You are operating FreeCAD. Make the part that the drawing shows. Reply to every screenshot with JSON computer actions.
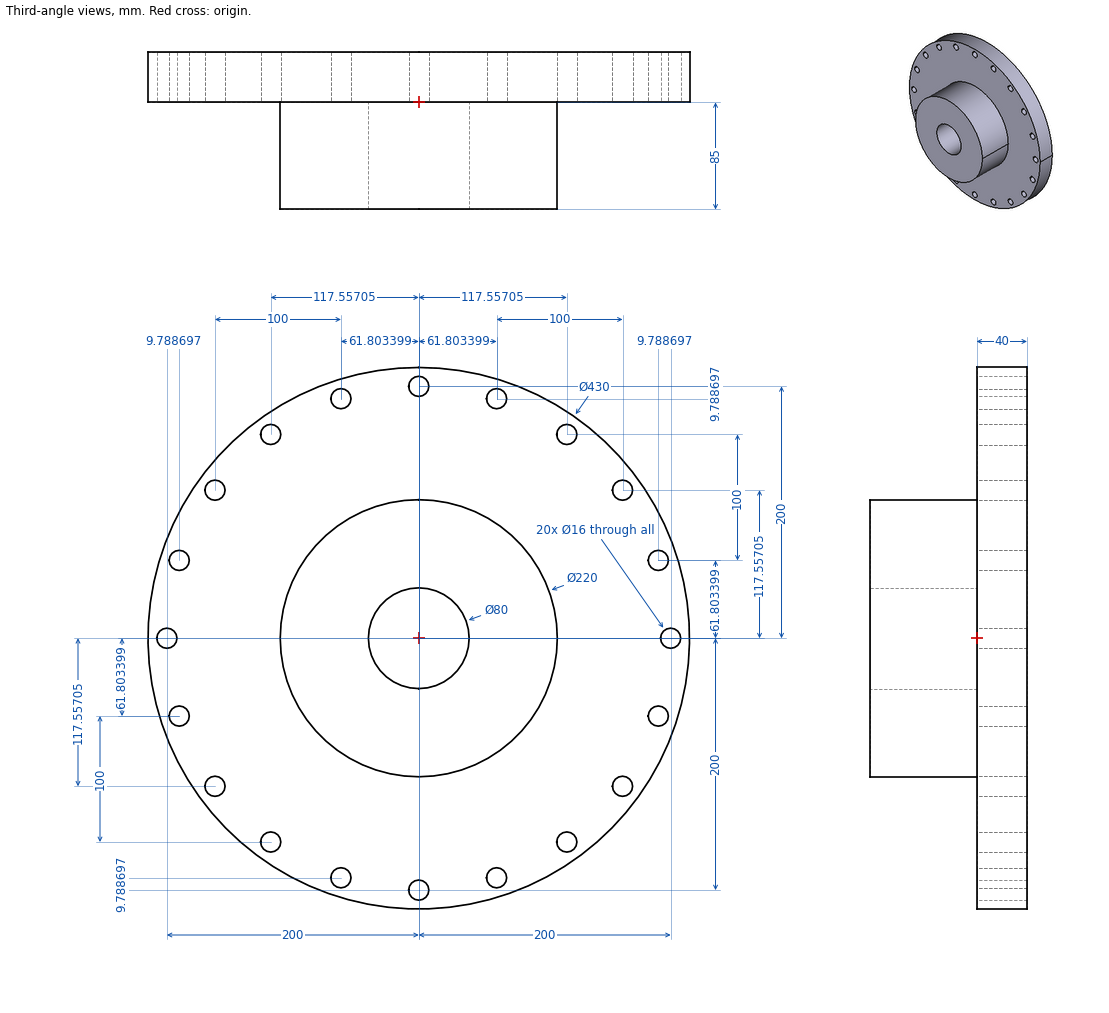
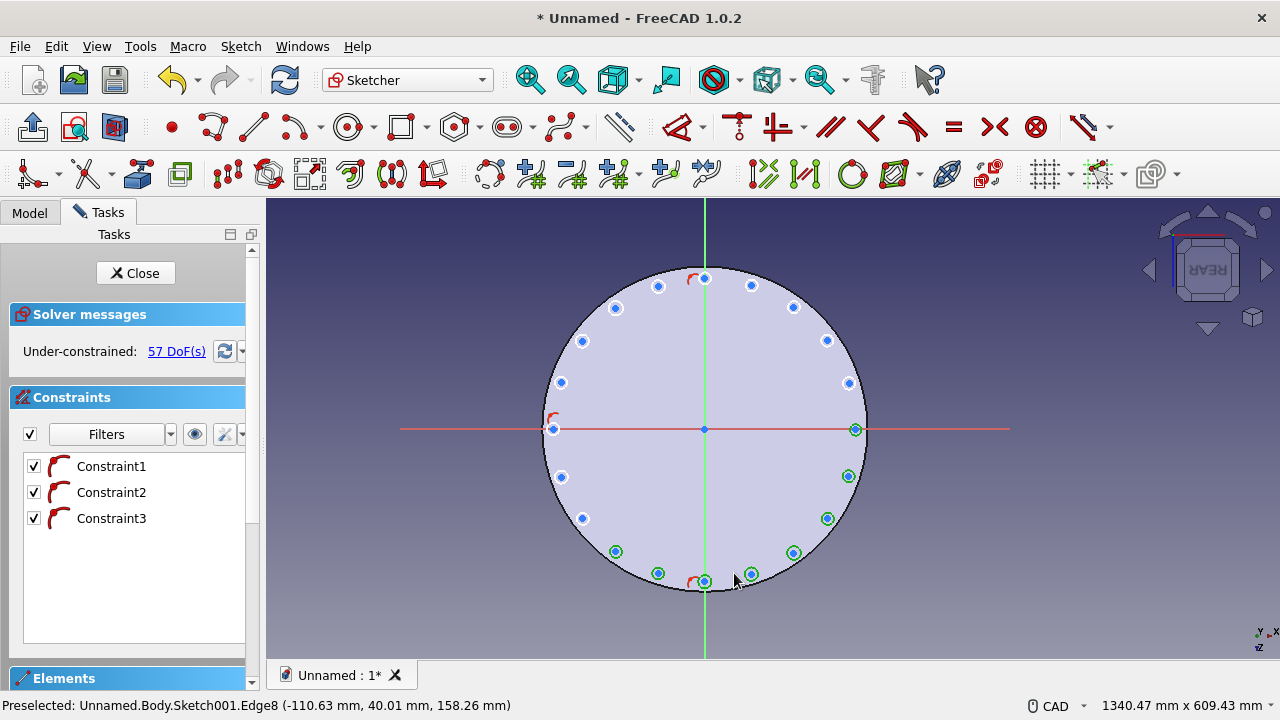
{"action": "scroll", "coordinate": [587, 515], "scroll_direction": "up", "scroll_amount": 5}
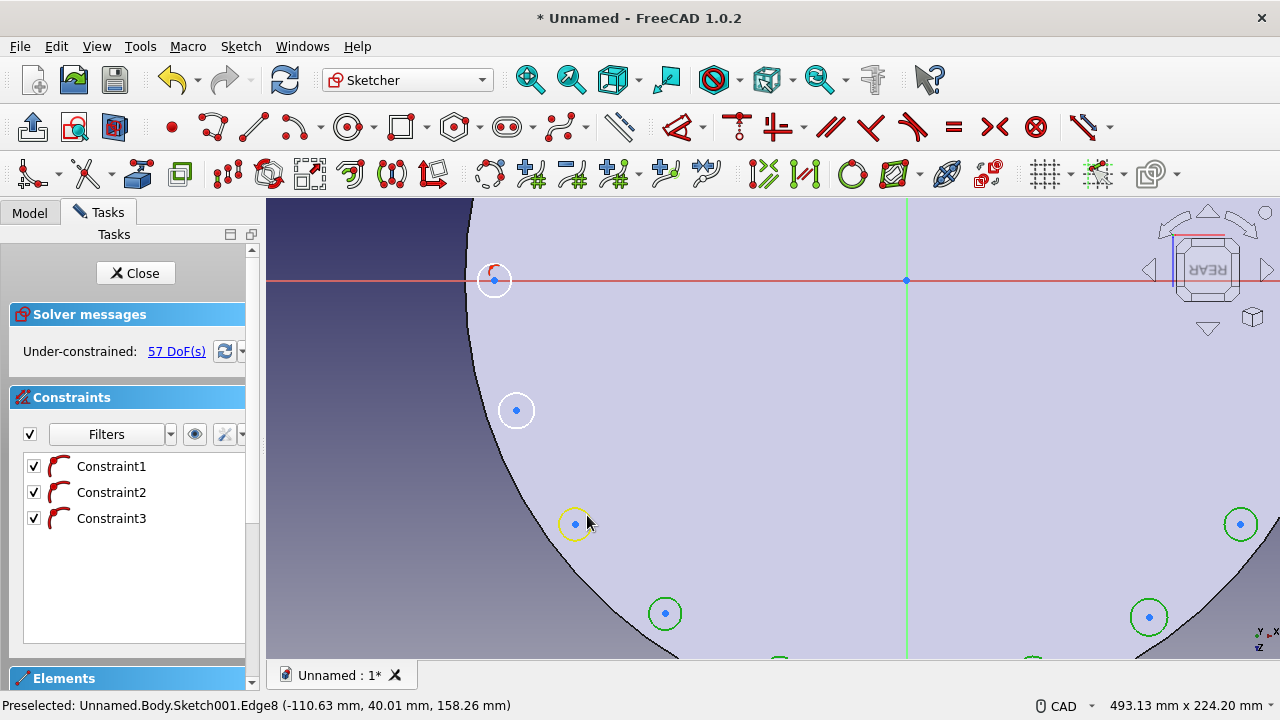
{"action": "left_click", "coordinate": [587, 513]}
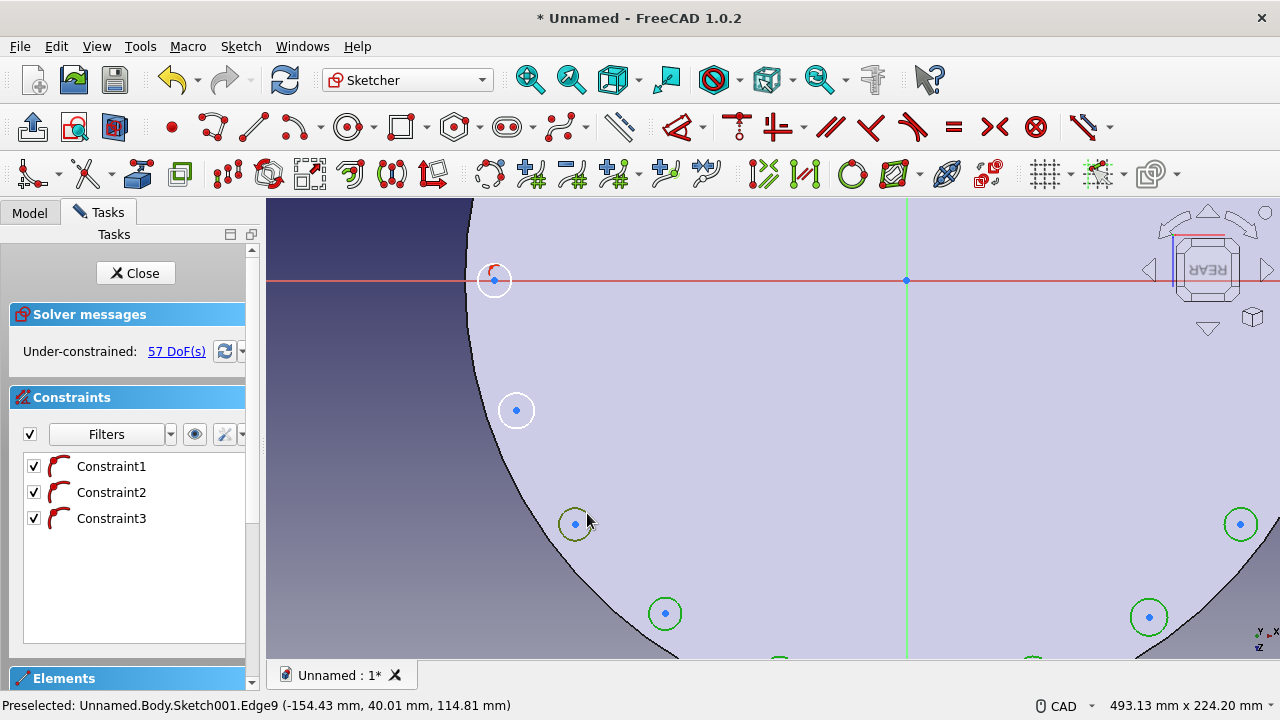
{"action": "left_click", "coordinate": [529, 398]}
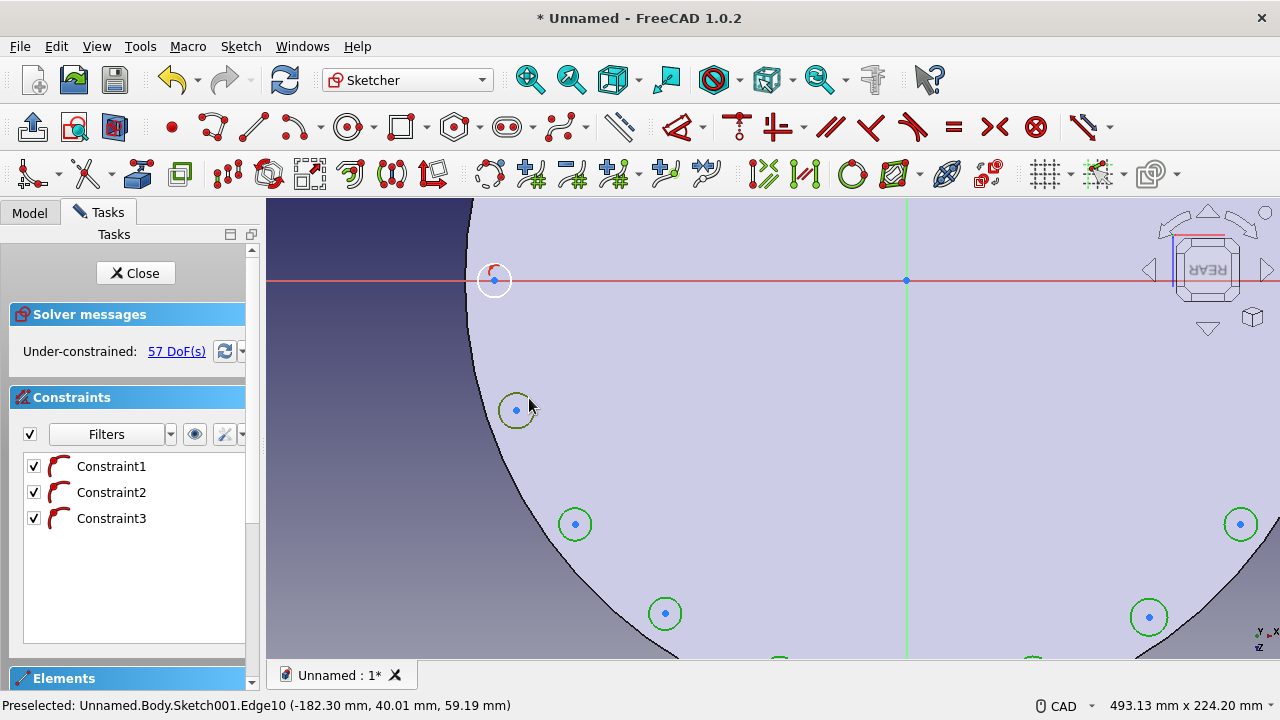
{"action": "left_click", "coordinate": [506, 269]}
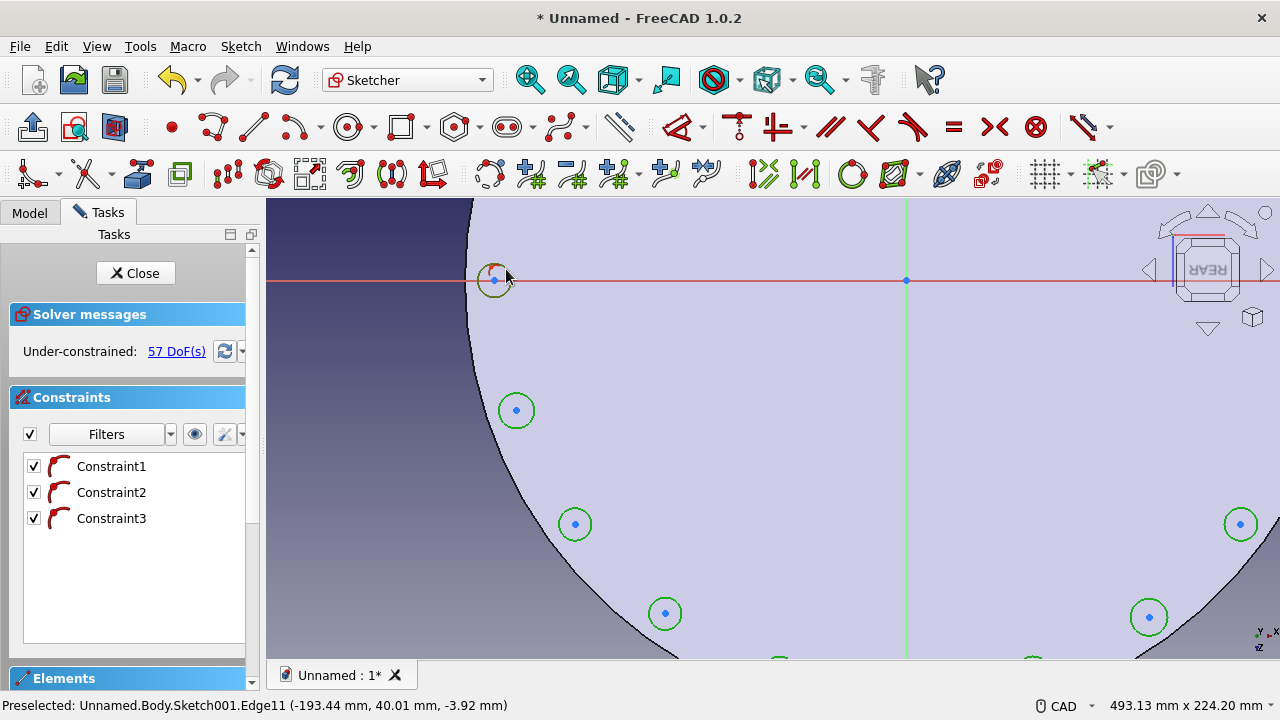
{"action": "scroll", "coordinate": [587, 515], "scroll_direction": "down", "scroll_amount": 5}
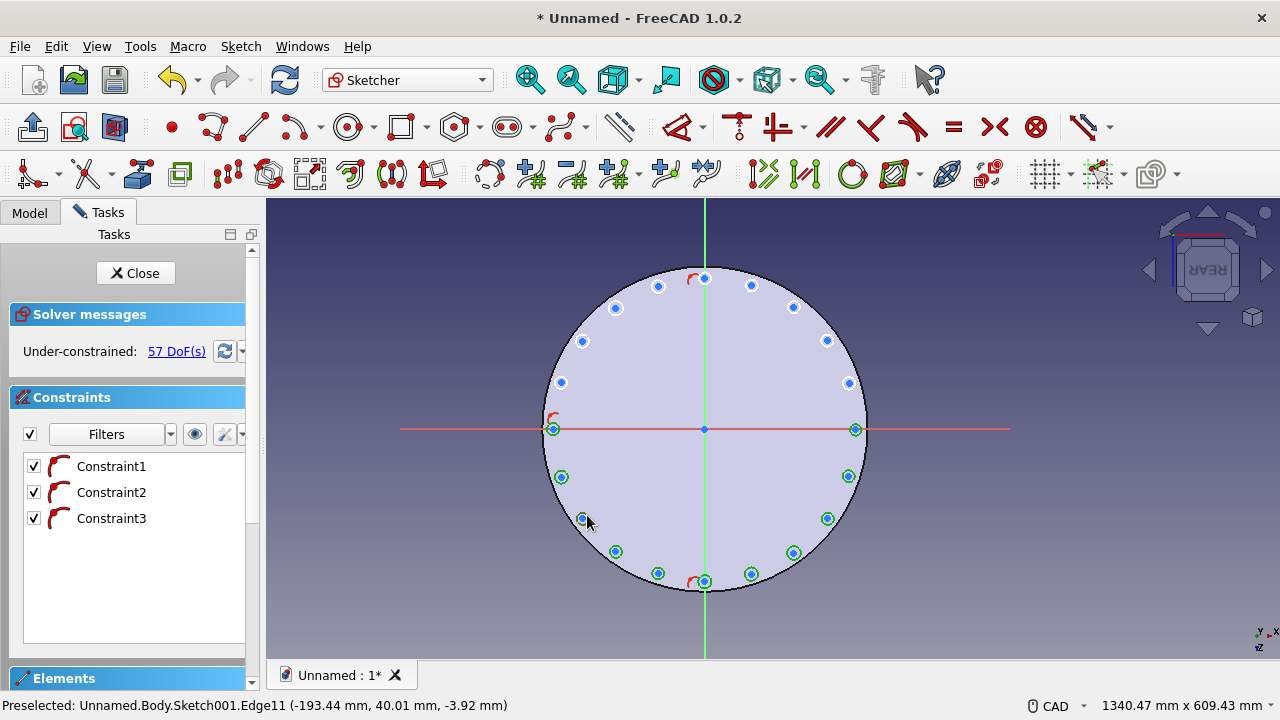
{"action": "scroll", "coordinate": [565, 379], "scroll_direction": "up", "scroll_amount": 5}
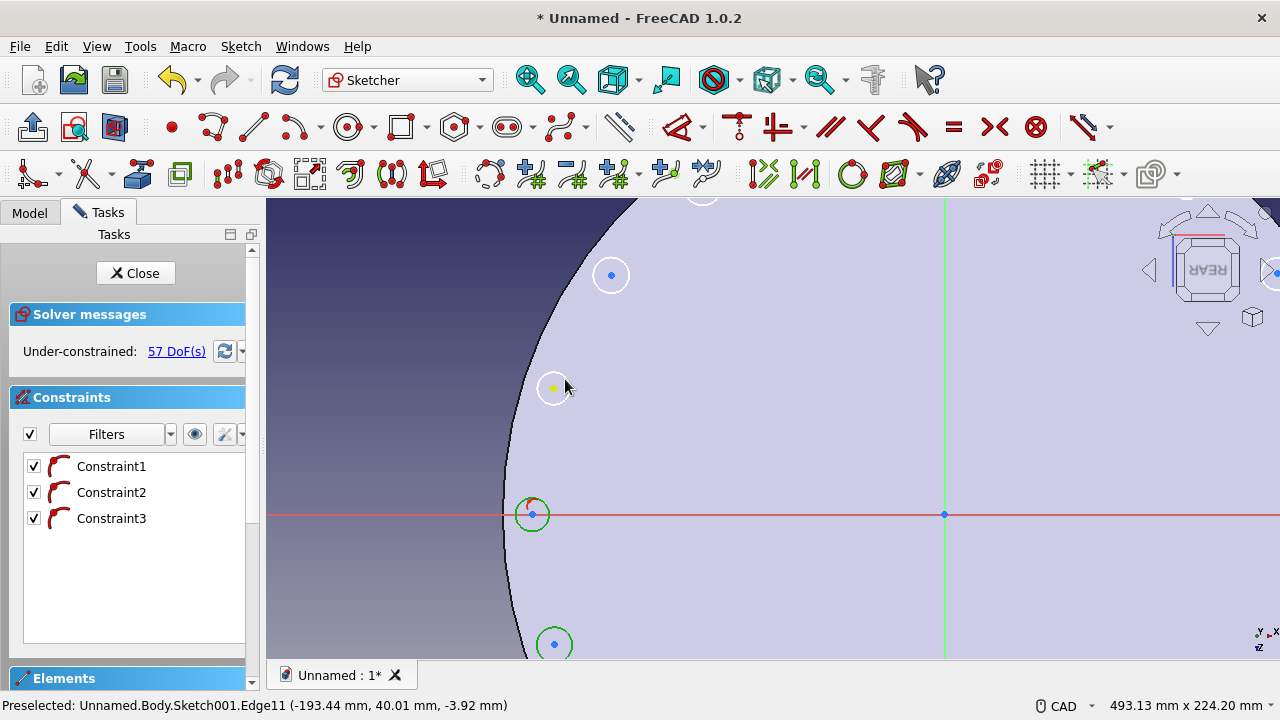
{"action": "left_click", "coordinate": [565, 377]}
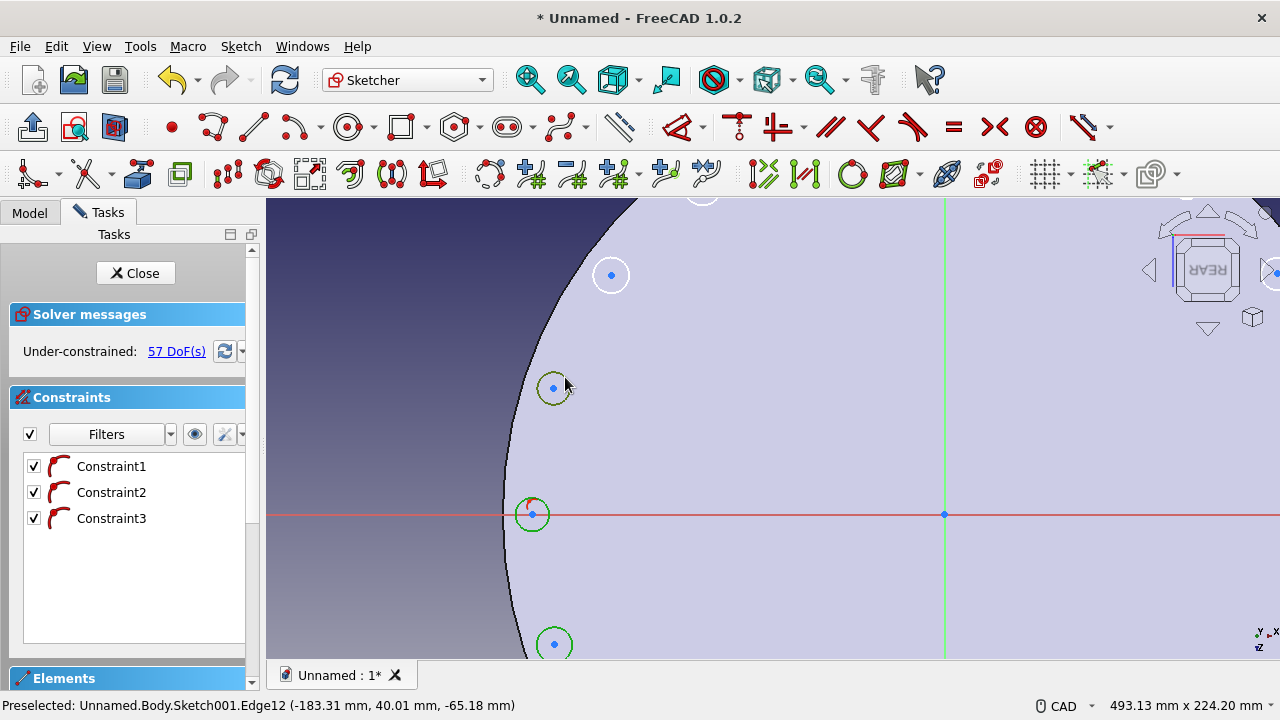
{"action": "left_click", "coordinate": [624, 263]}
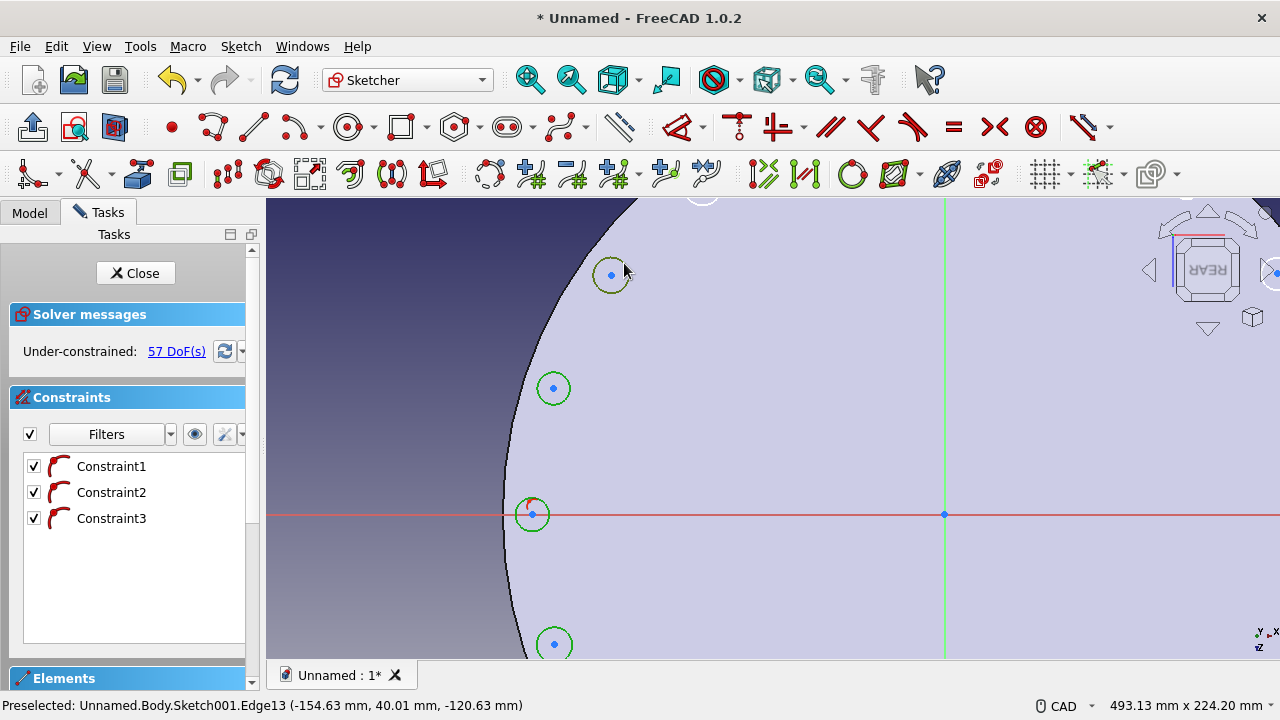
{"action": "scroll", "coordinate": [565, 378], "scroll_direction": "down", "scroll_amount": 5}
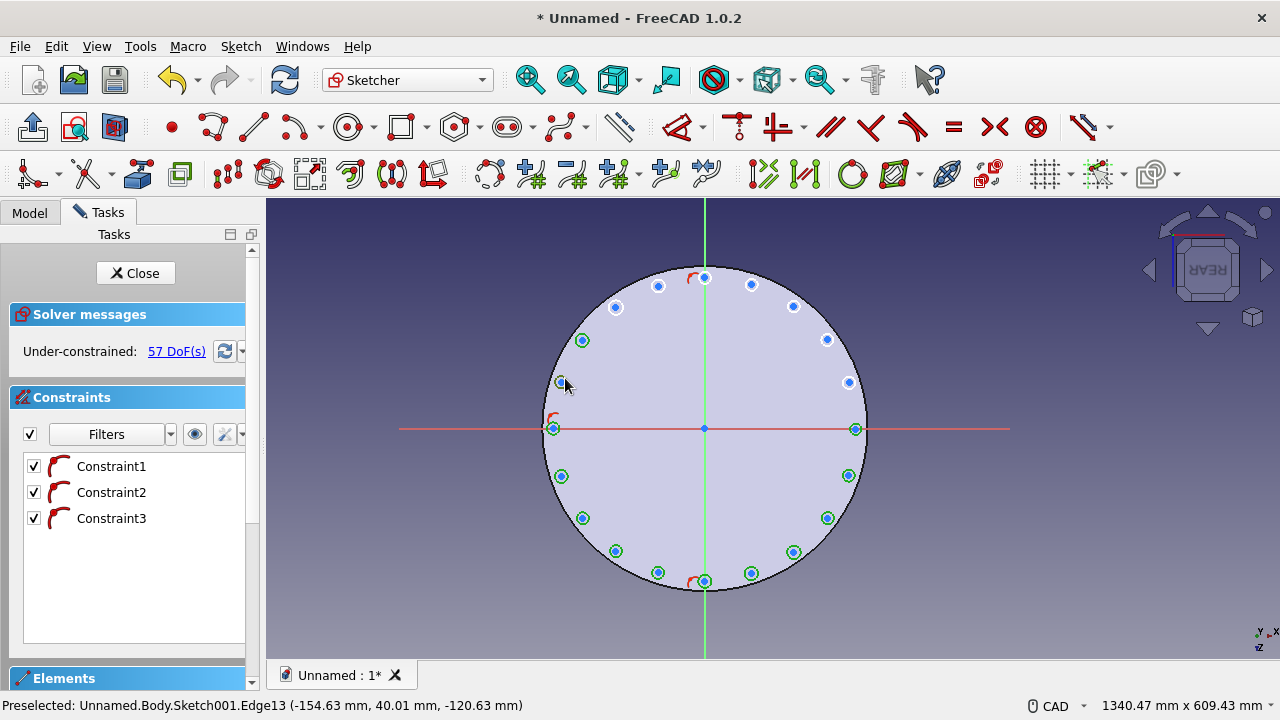
{"action": "scroll", "coordinate": [621, 302], "scroll_direction": "up", "scroll_amount": 4}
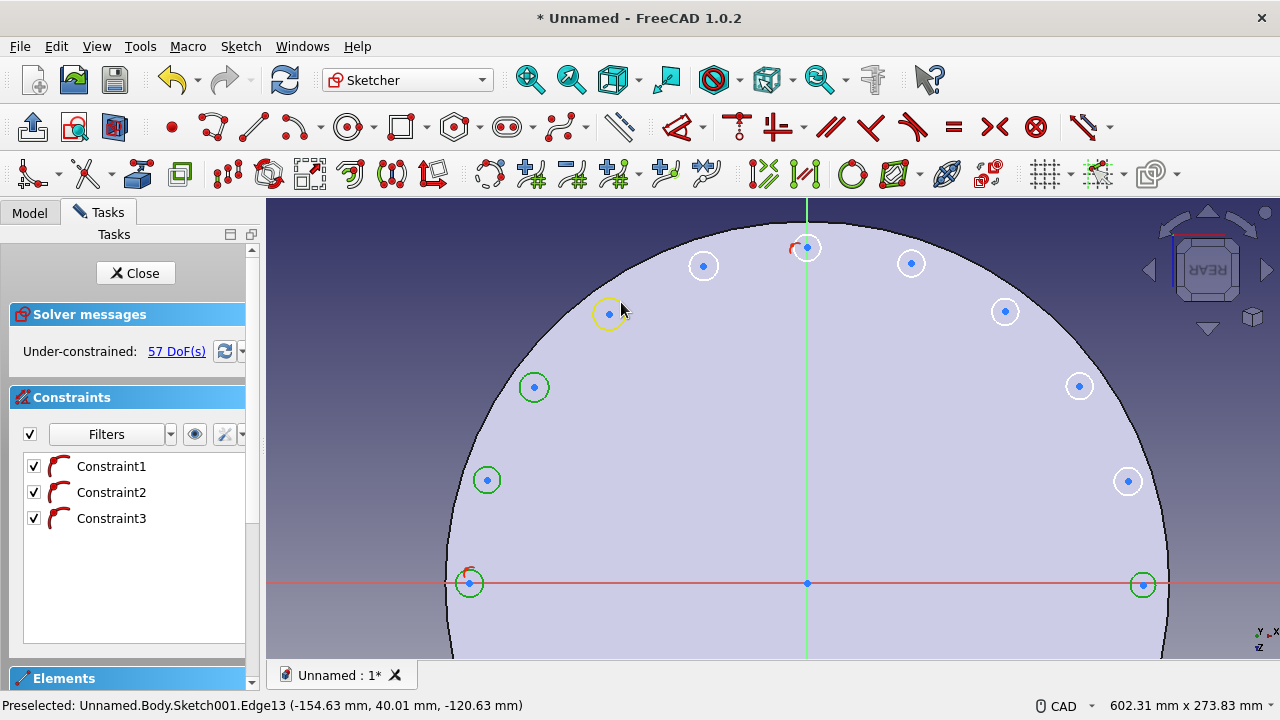
{"action": "left_click", "coordinate": [620, 303]}